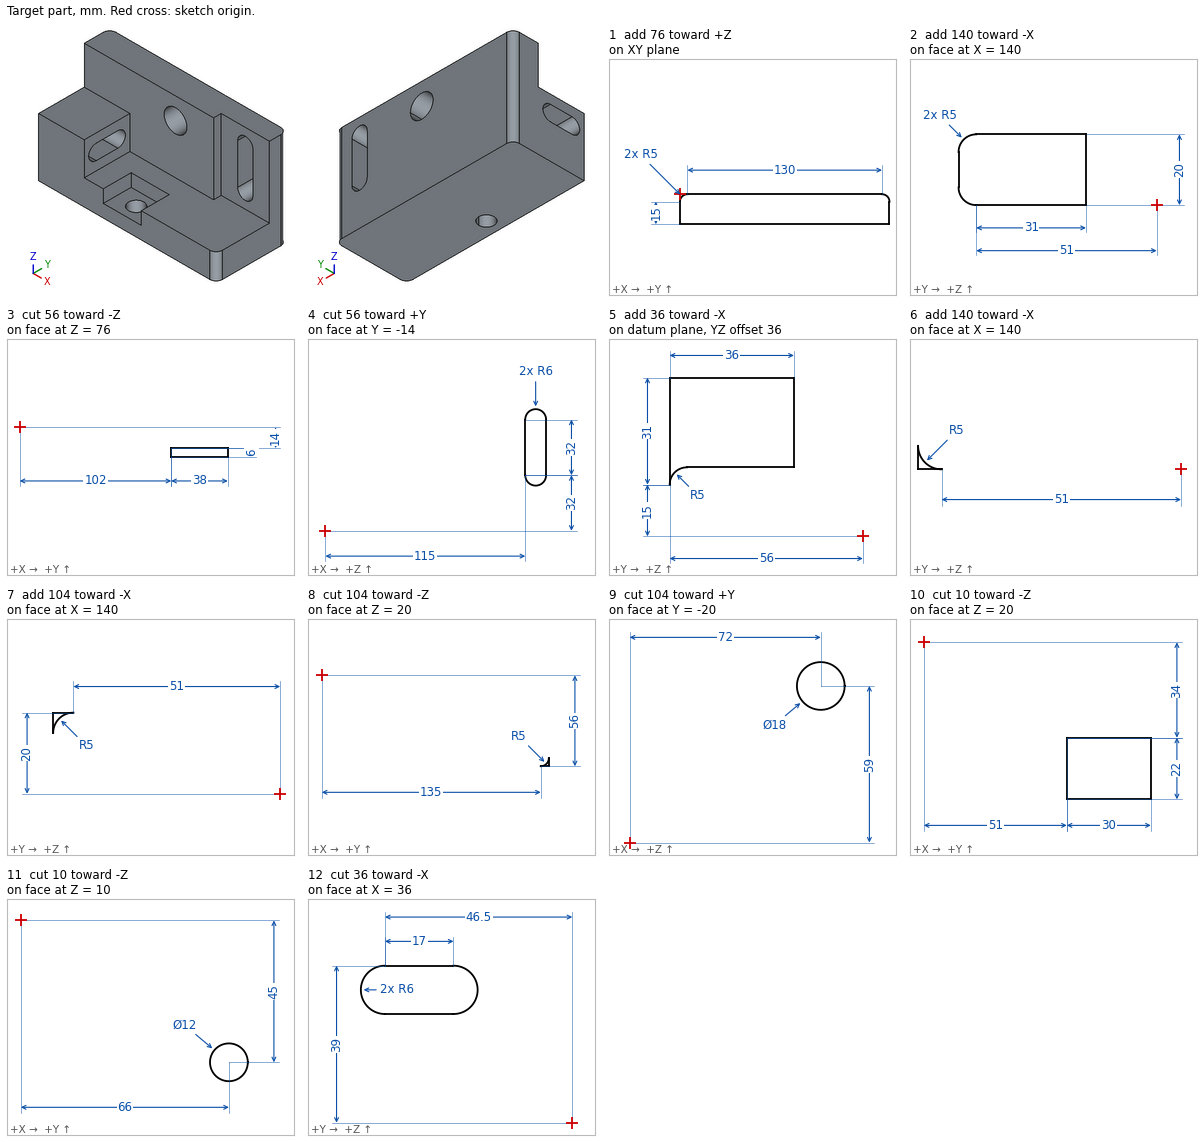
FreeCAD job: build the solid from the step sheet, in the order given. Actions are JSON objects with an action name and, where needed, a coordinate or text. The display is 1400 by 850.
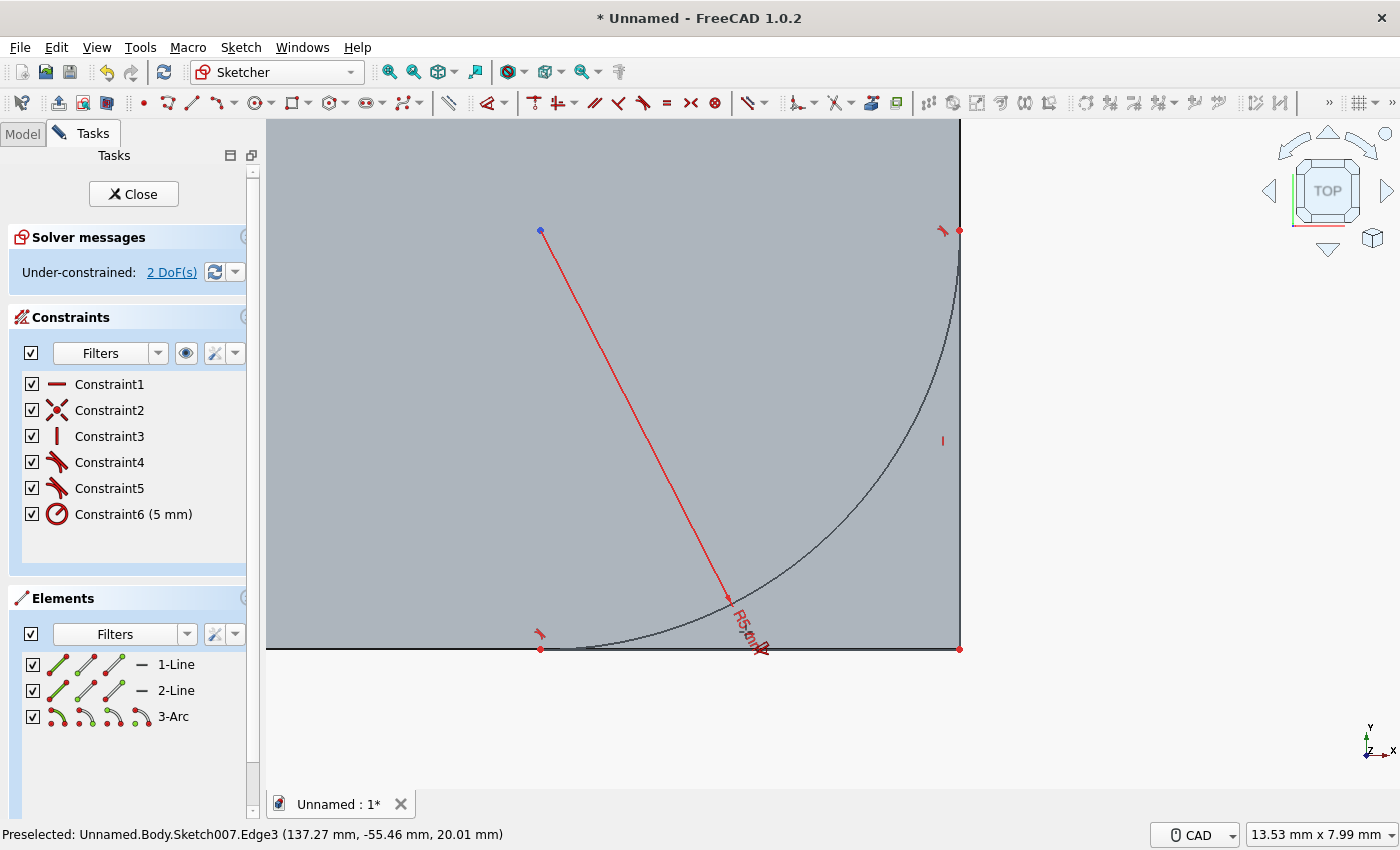
{"action": "left_click", "coordinate": [541, 650]}
{"action": "left_click", "coordinate": [575, 398]}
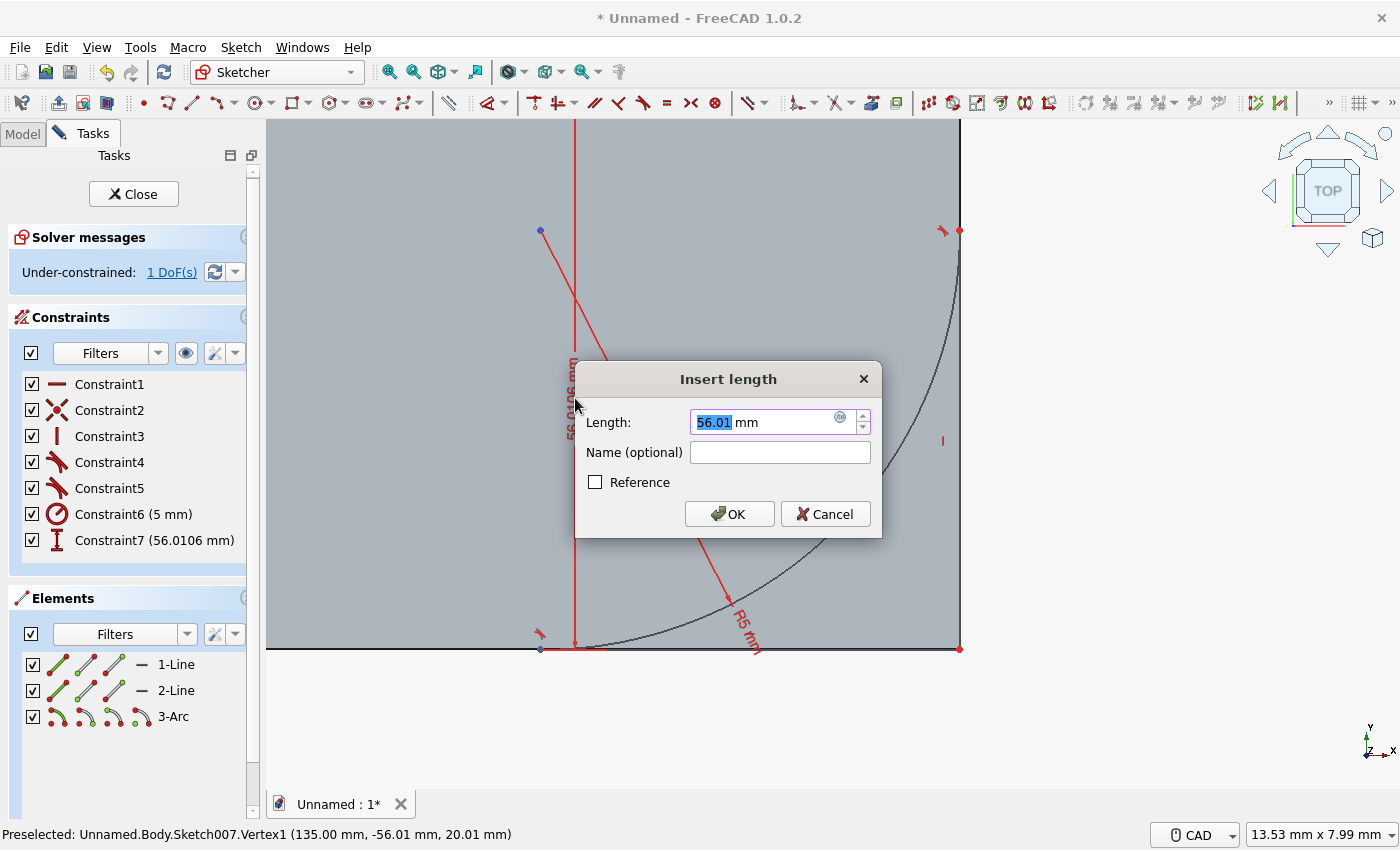
{"action": "type", "text": "56"}
{"action": "key", "text": "Return"}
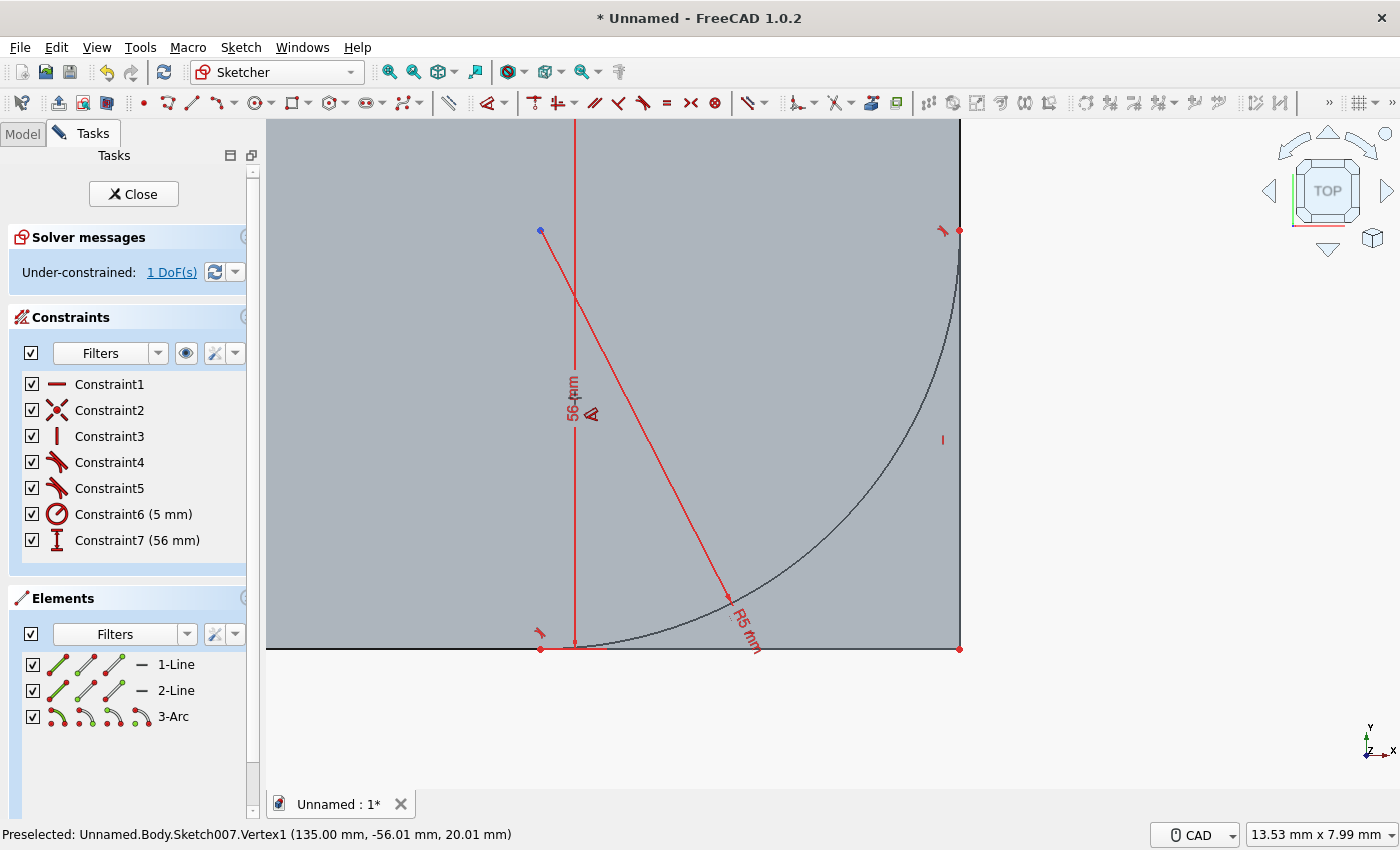
{"action": "left_click", "coordinate": [541, 649]}
{"action": "left_click", "coordinate": [417, 683]}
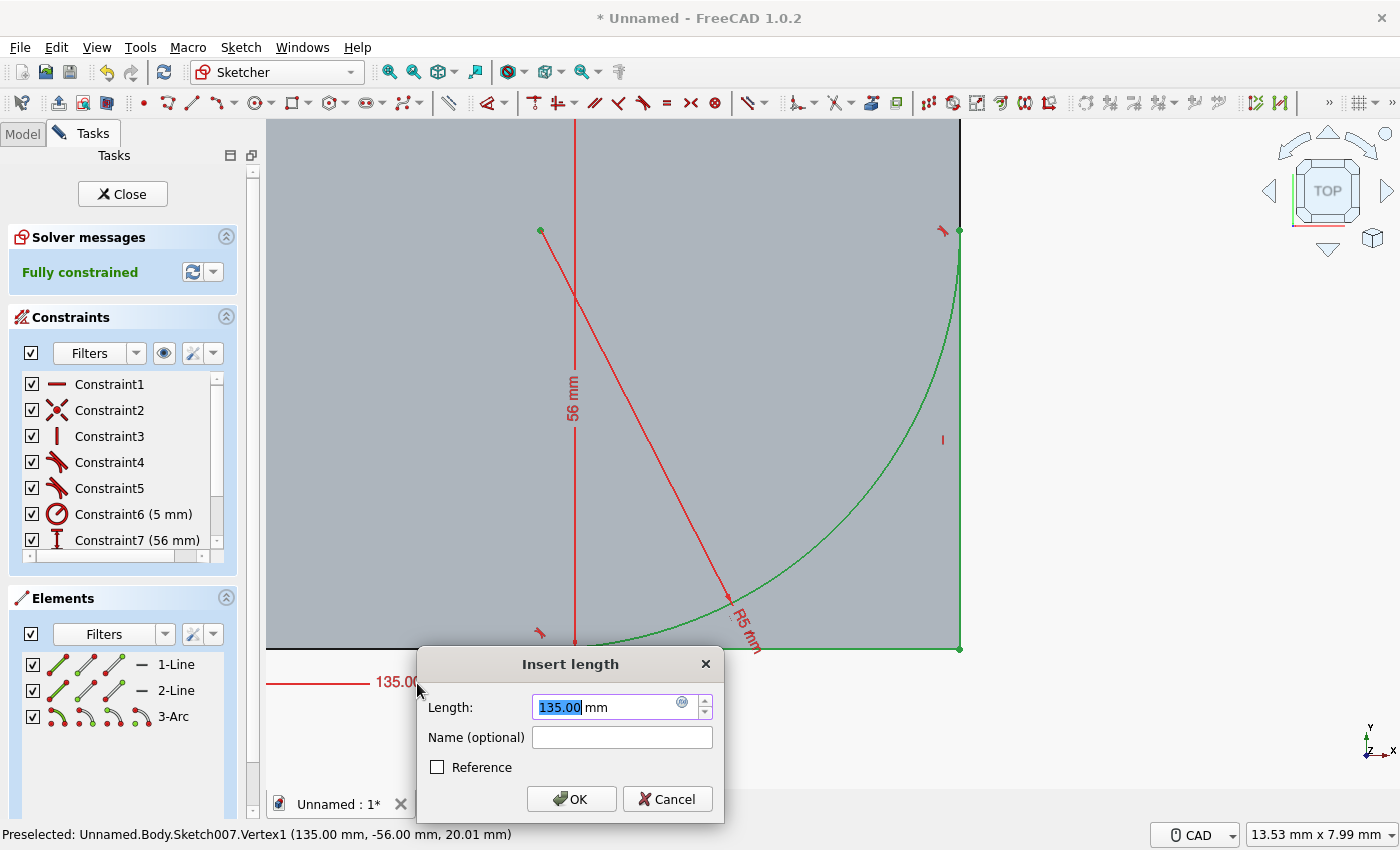
{"action": "type", "text": "135"}
{"action": "key", "text": "Return"}
{"action": "key", "text": "Escape"}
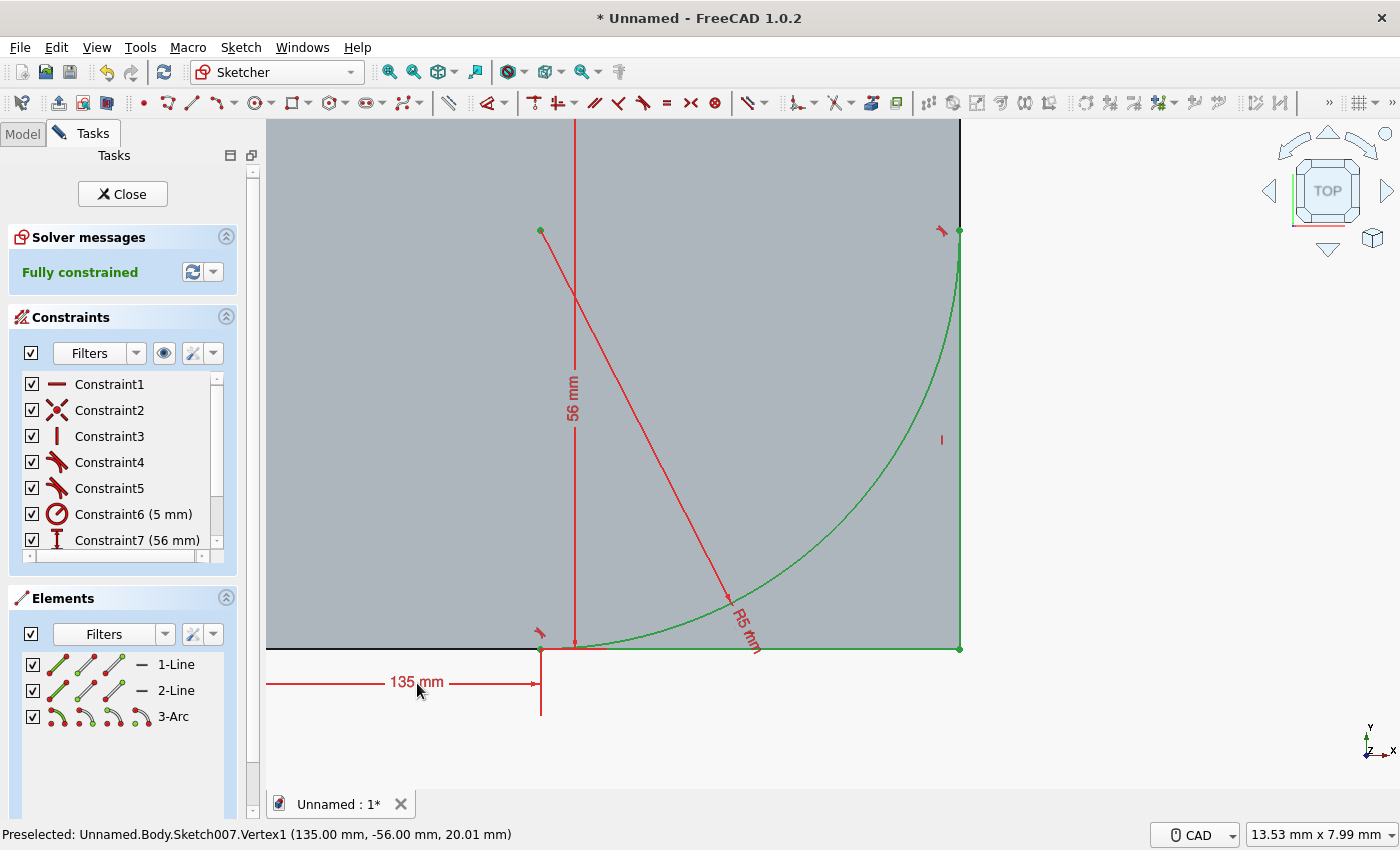
{"action": "left_click", "coordinate": [123, 194]}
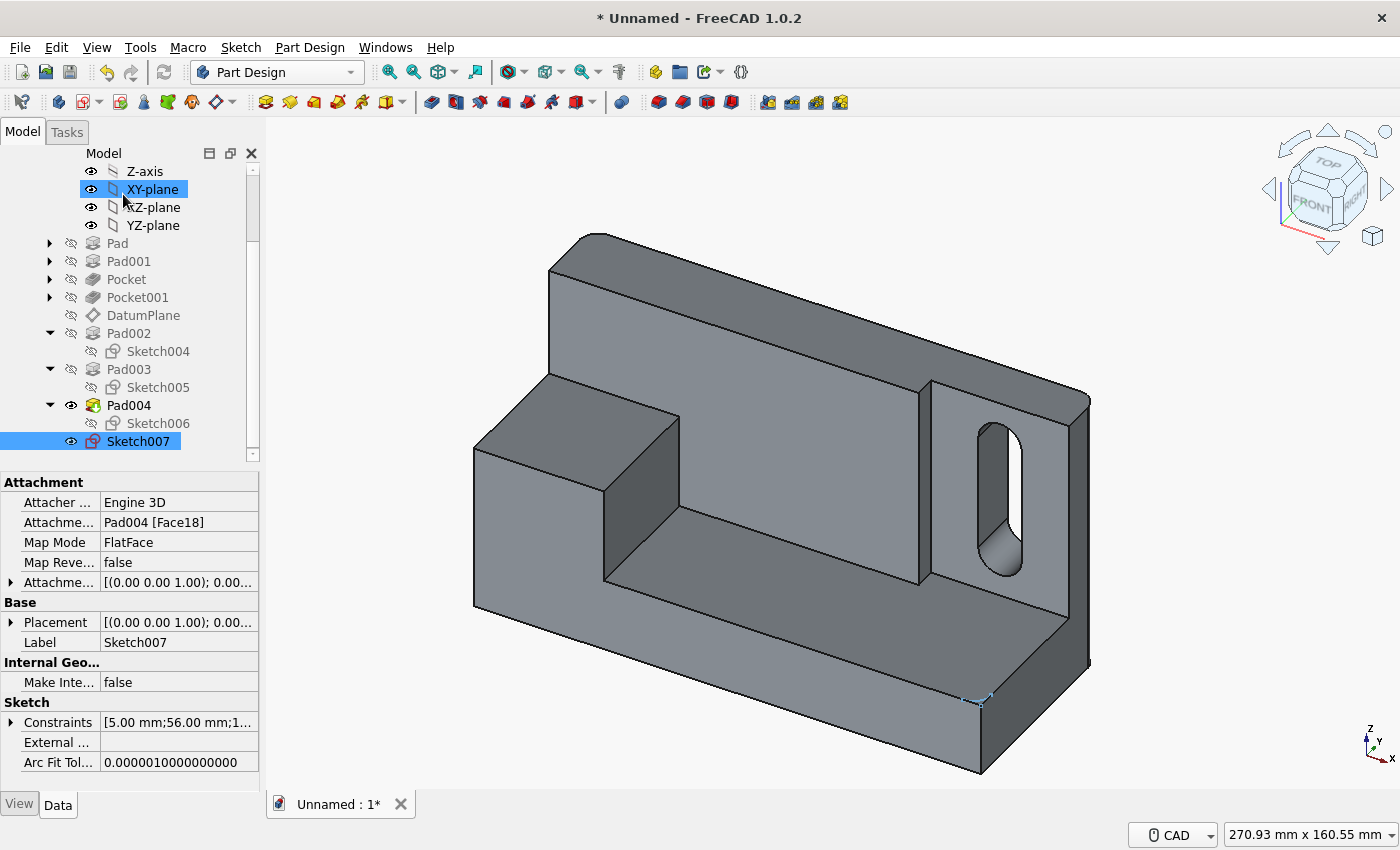
{"action": "left_click", "coordinate": [432, 102]}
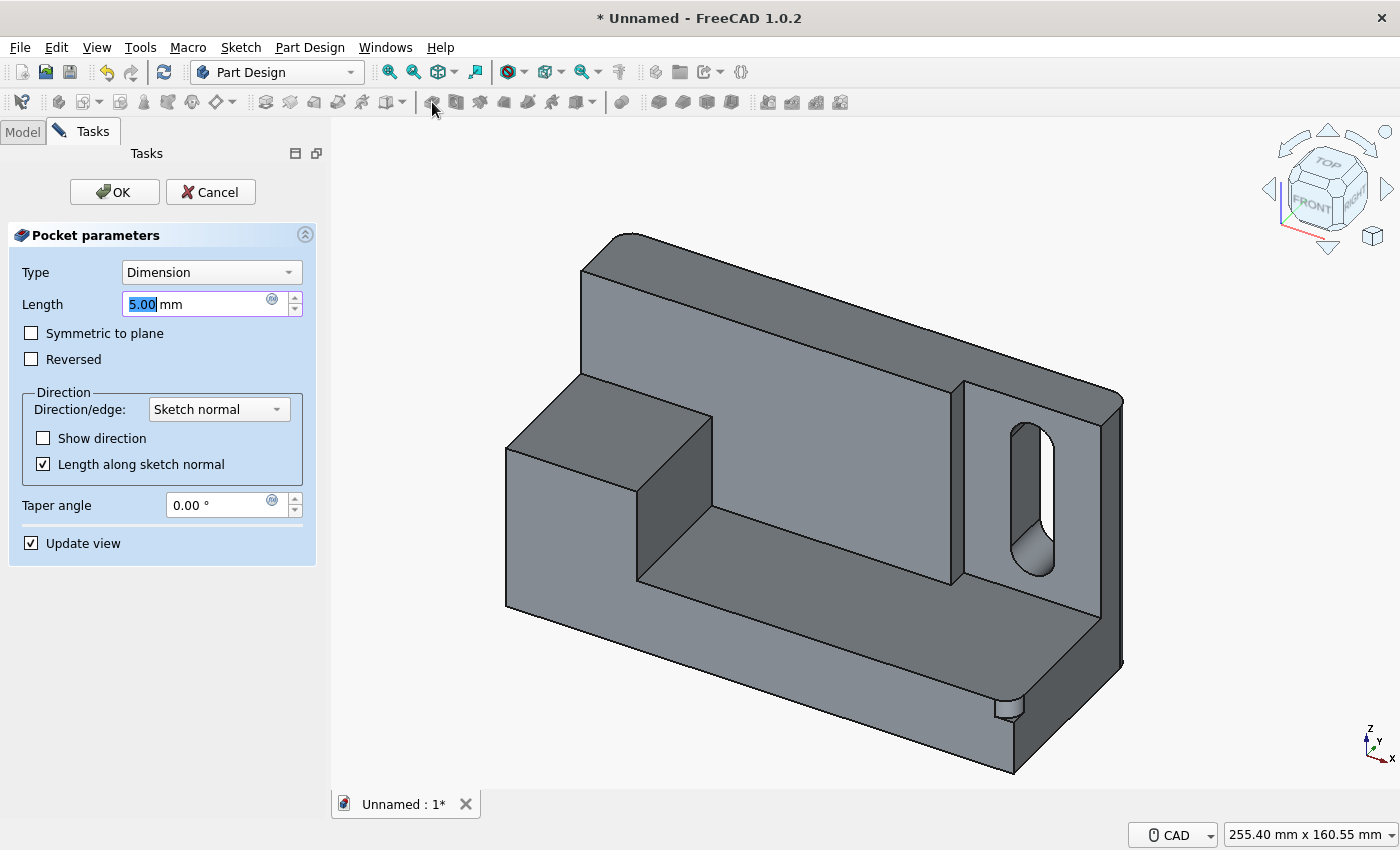
{"action": "type", "text": "104"}
{"action": "key", "text": "Tab"}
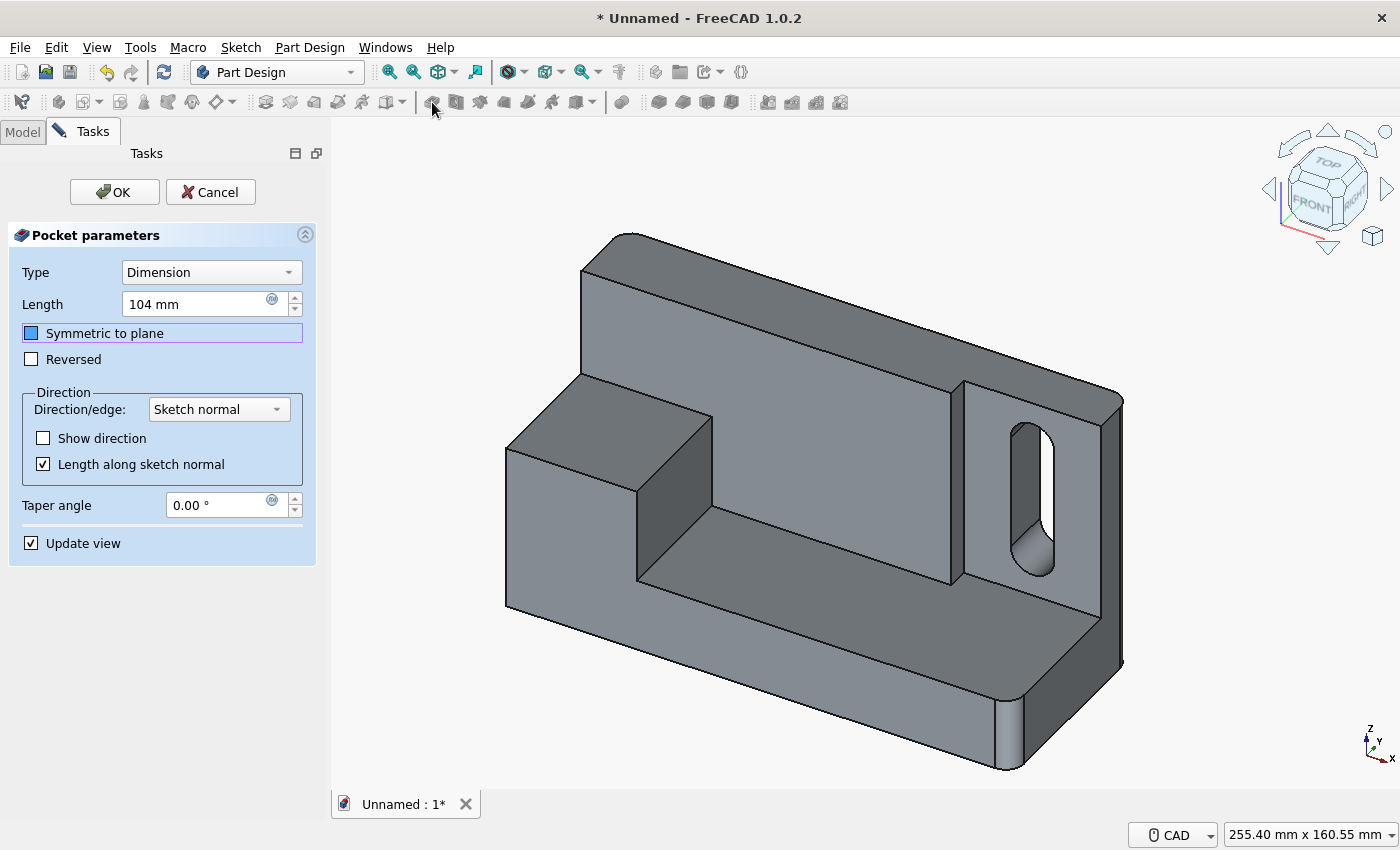
{"action": "left_click", "coordinate": [115, 192]}